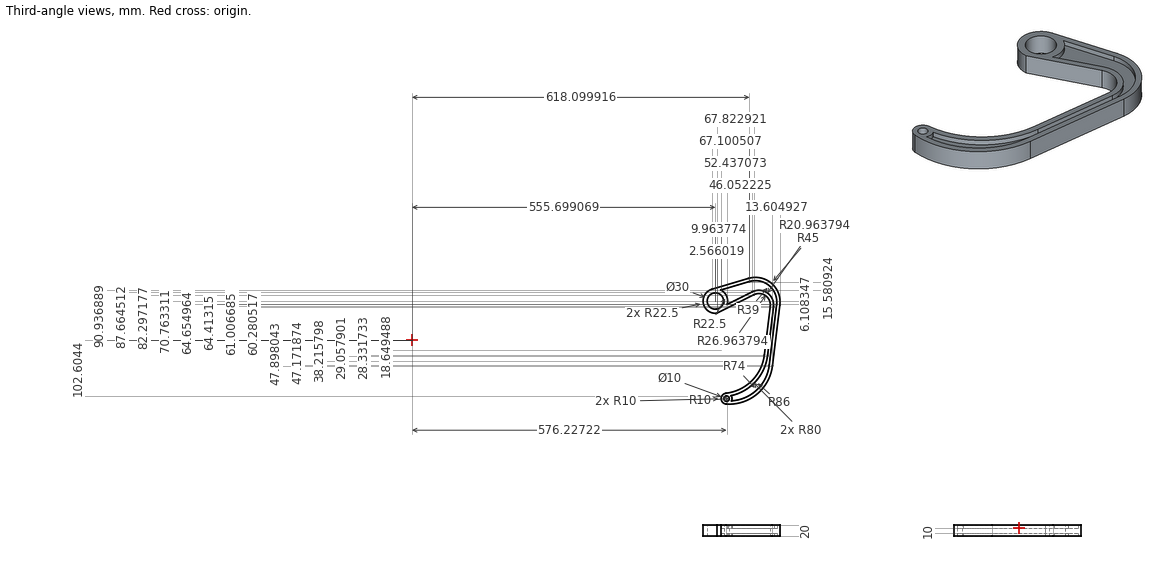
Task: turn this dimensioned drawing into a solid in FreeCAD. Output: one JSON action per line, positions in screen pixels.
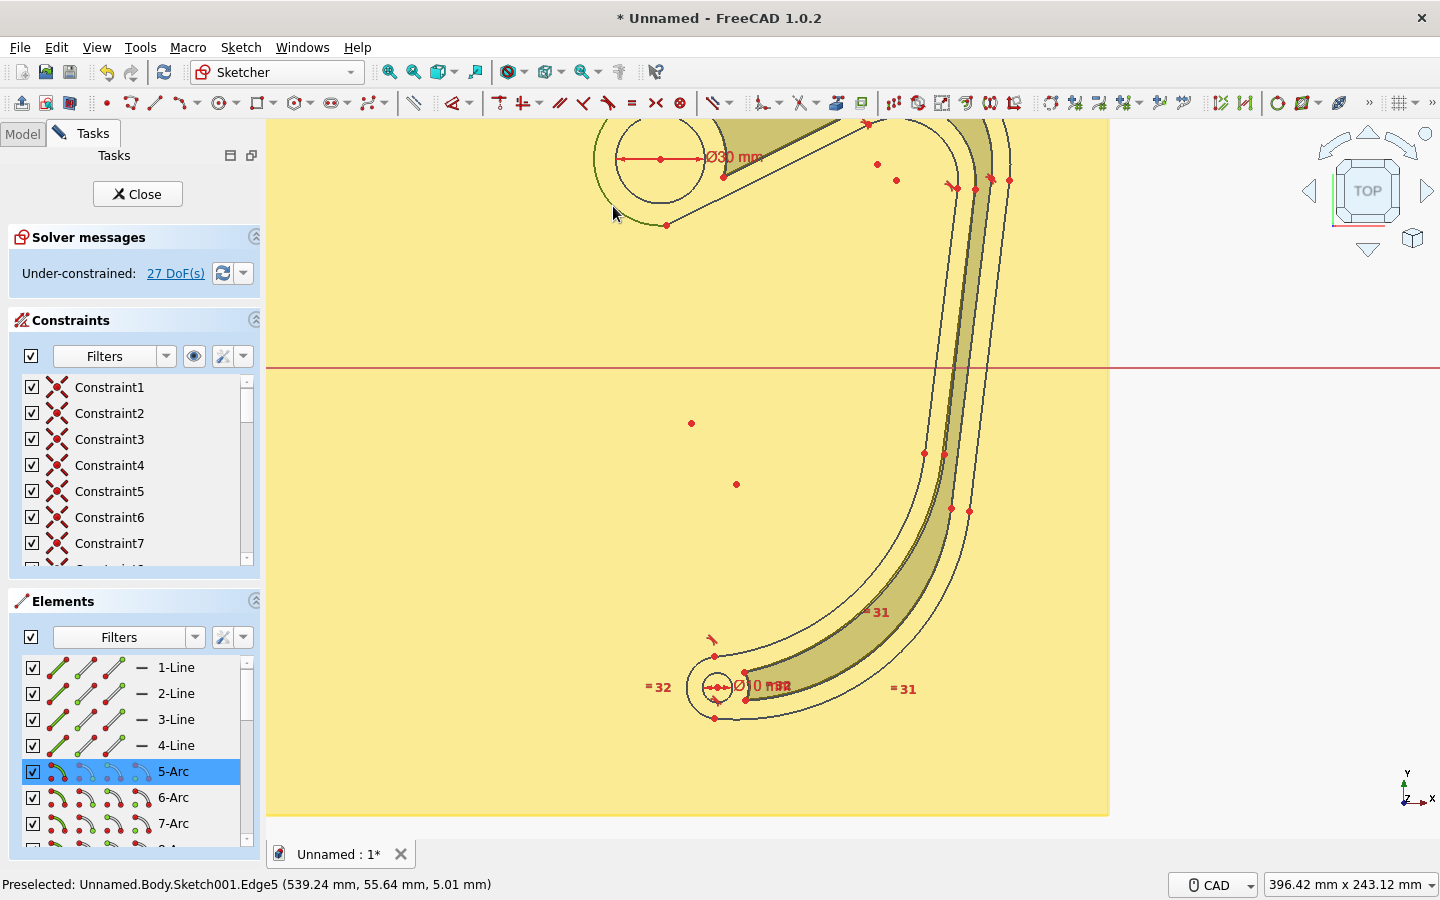
{"action": "left_click", "coordinate": [726, 150]}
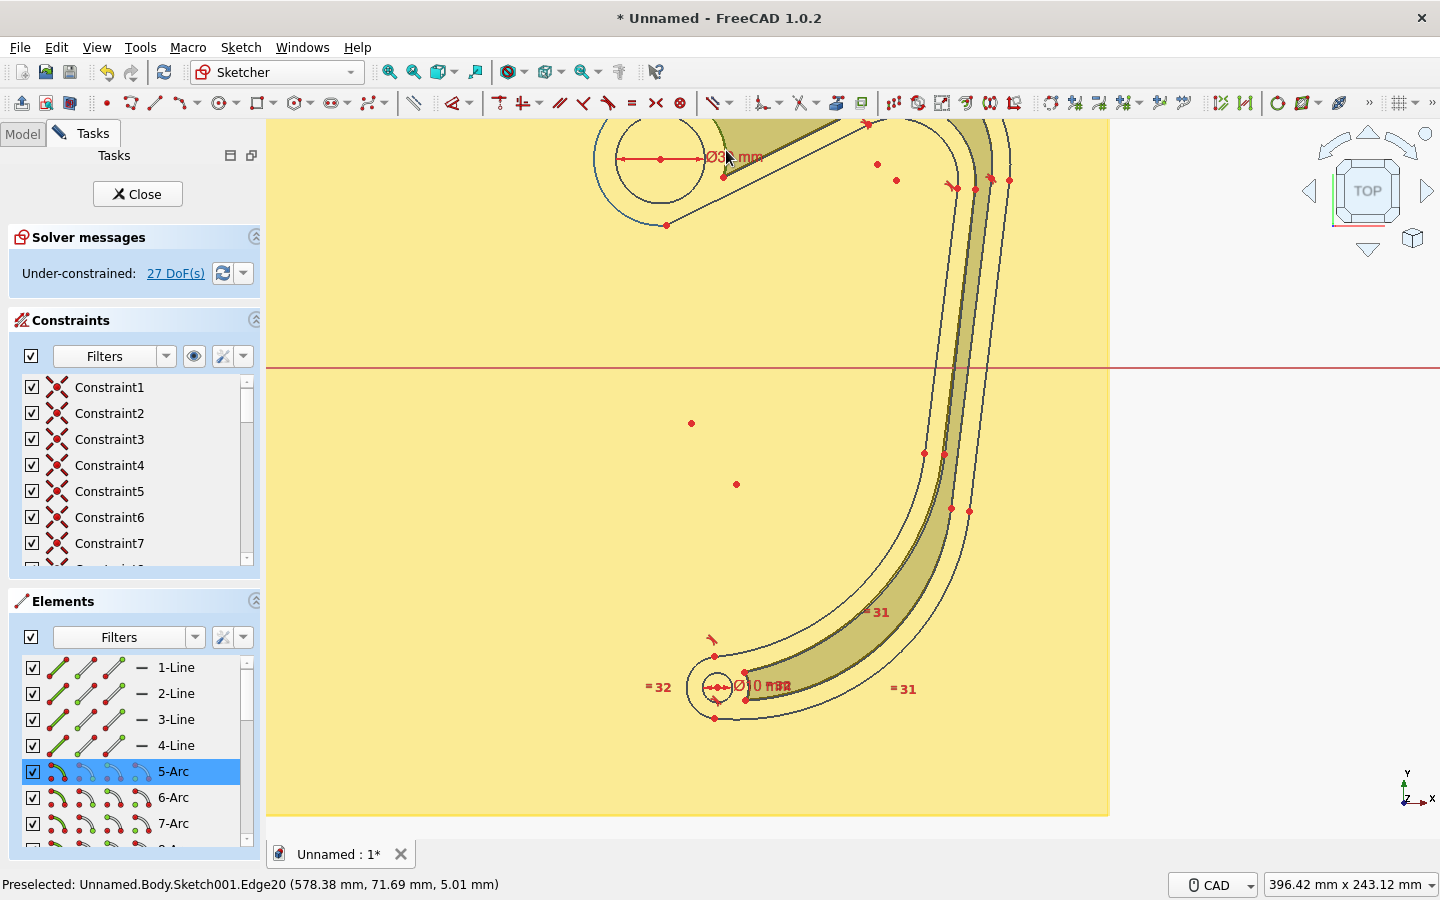
{"action": "key", "text": "e"}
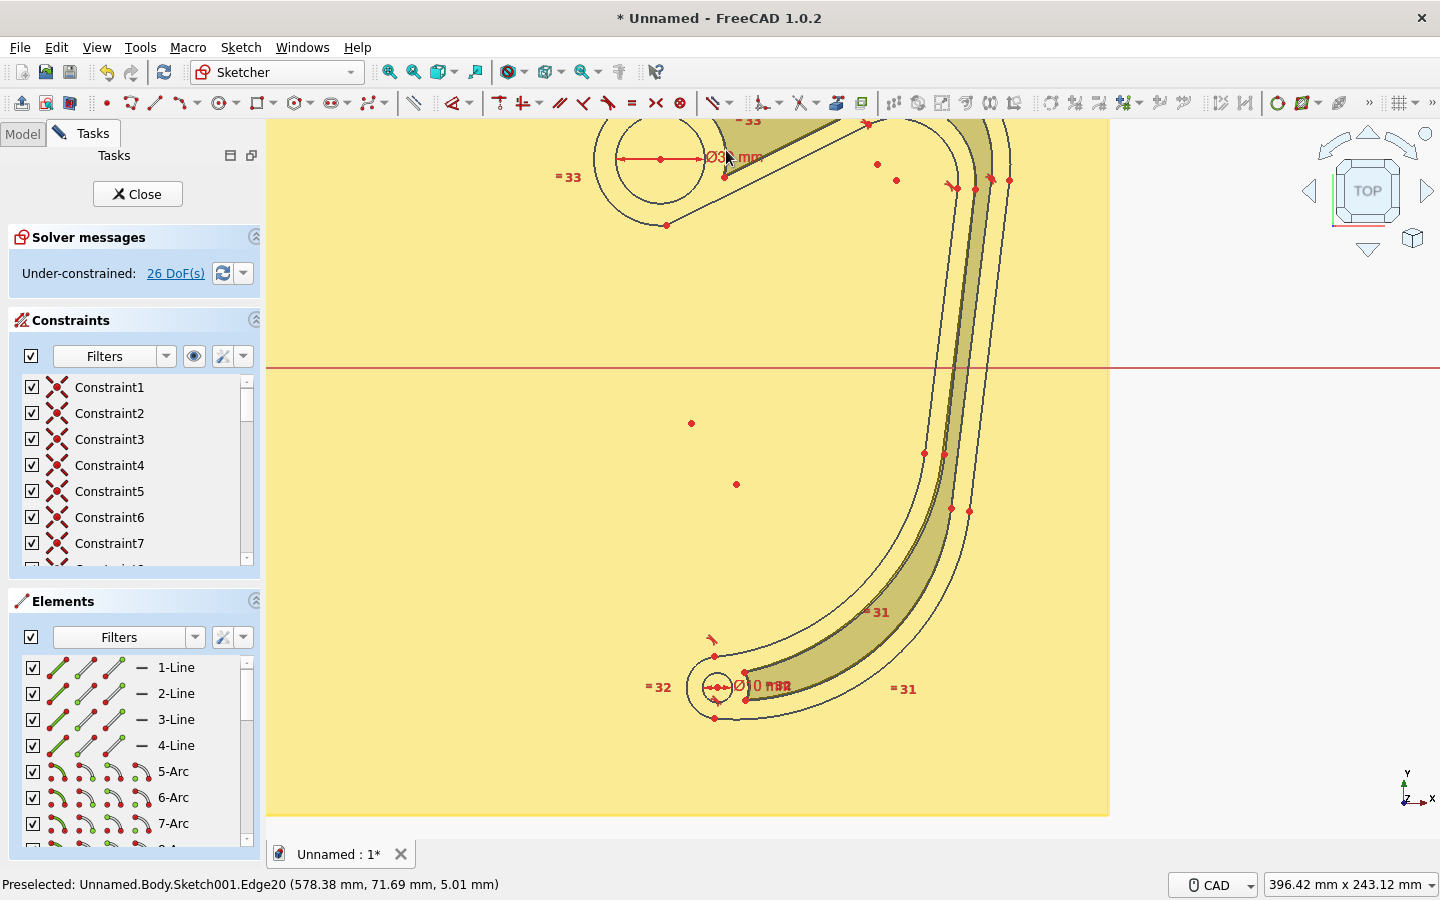
{"action": "left_click", "coordinate": [452, 104]}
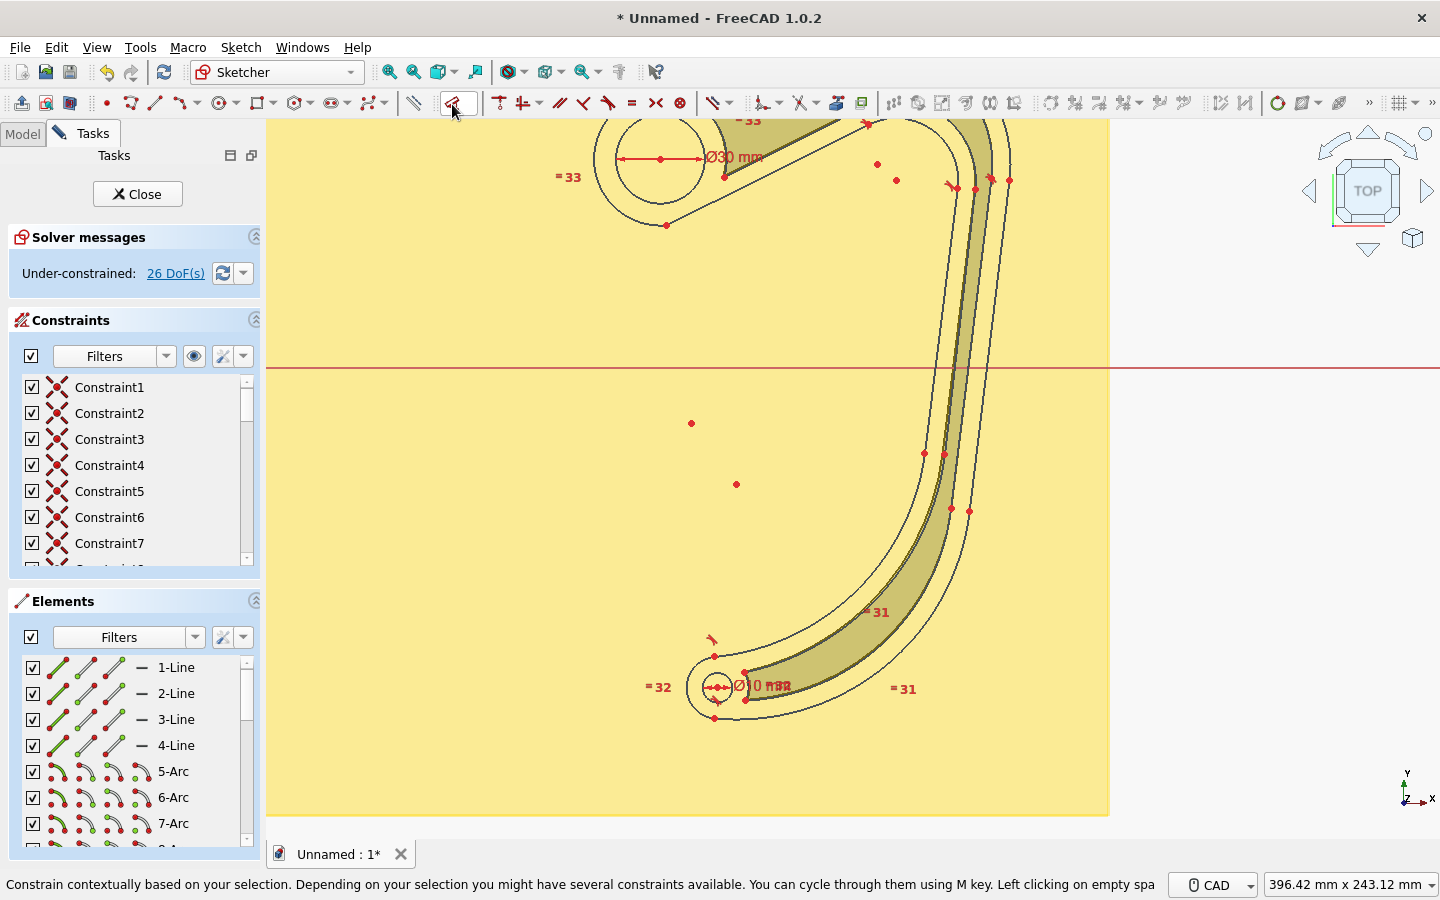
{"action": "left_click", "coordinate": [613, 206]}
{"action": "left_click", "coordinate": [590, 228]}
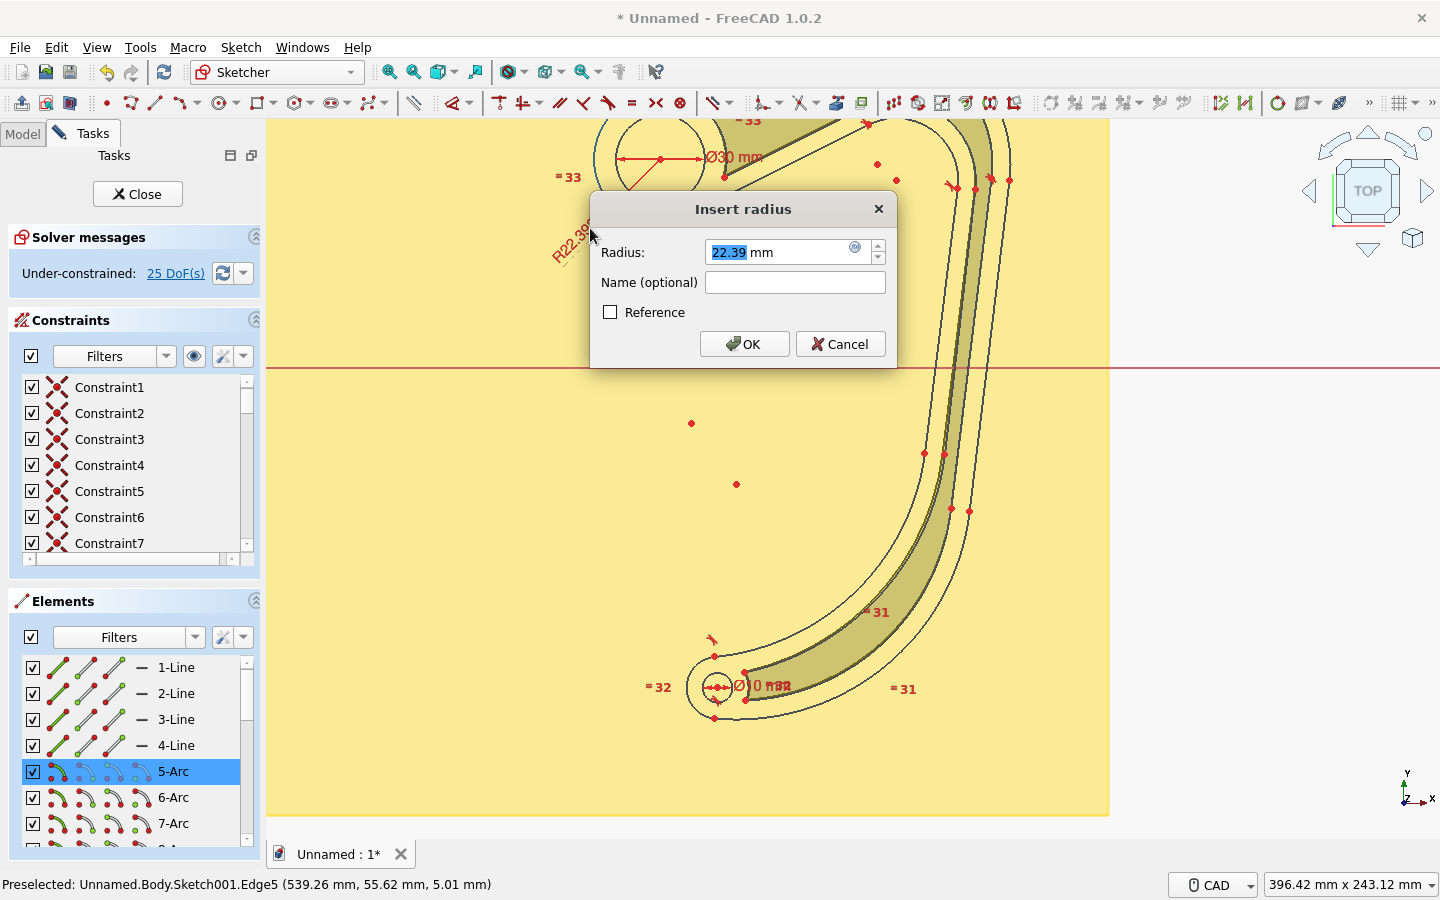
{"action": "type", "text": "22.5"}
{"action": "key", "text": "Return"}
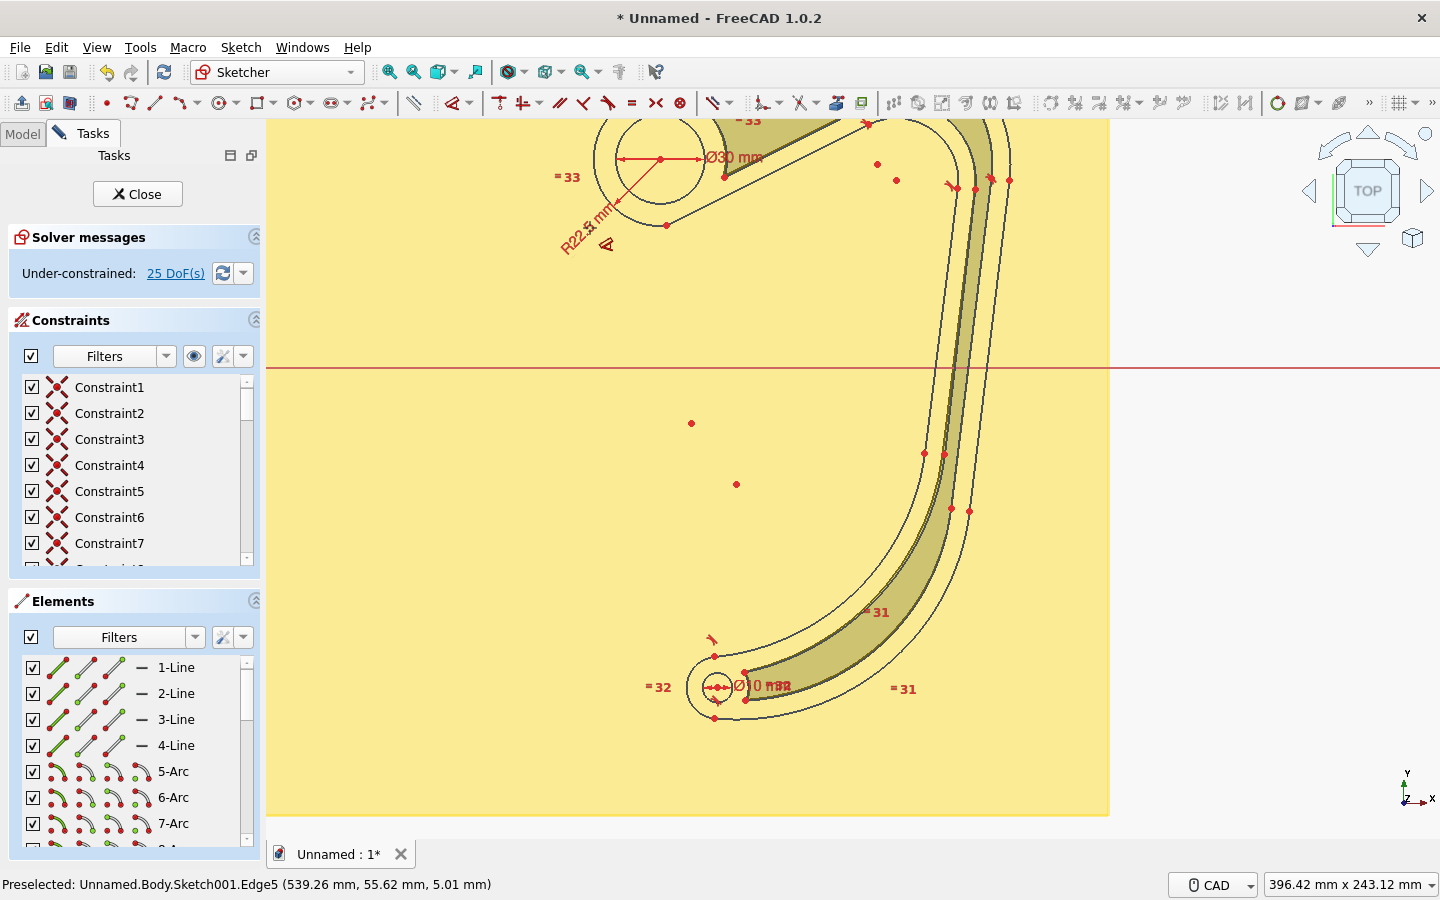
{"action": "left_click", "coordinate": [950, 149]}
{"action": "left_click", "coordinate": [815, 228]}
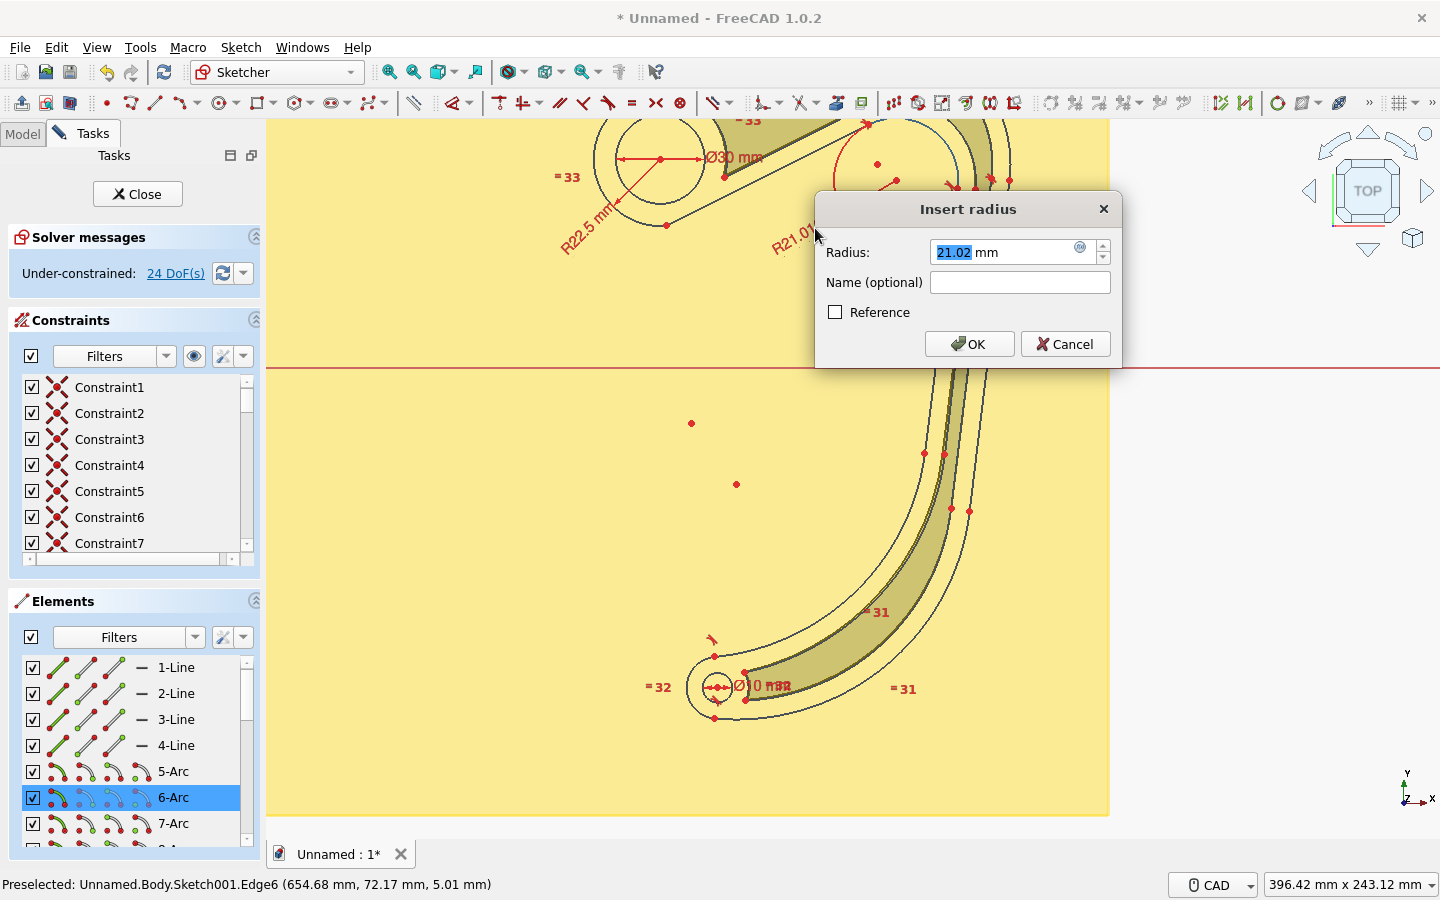
{"action": "type", "text": "20.963794"}
{"action": "key", "text": "Return"}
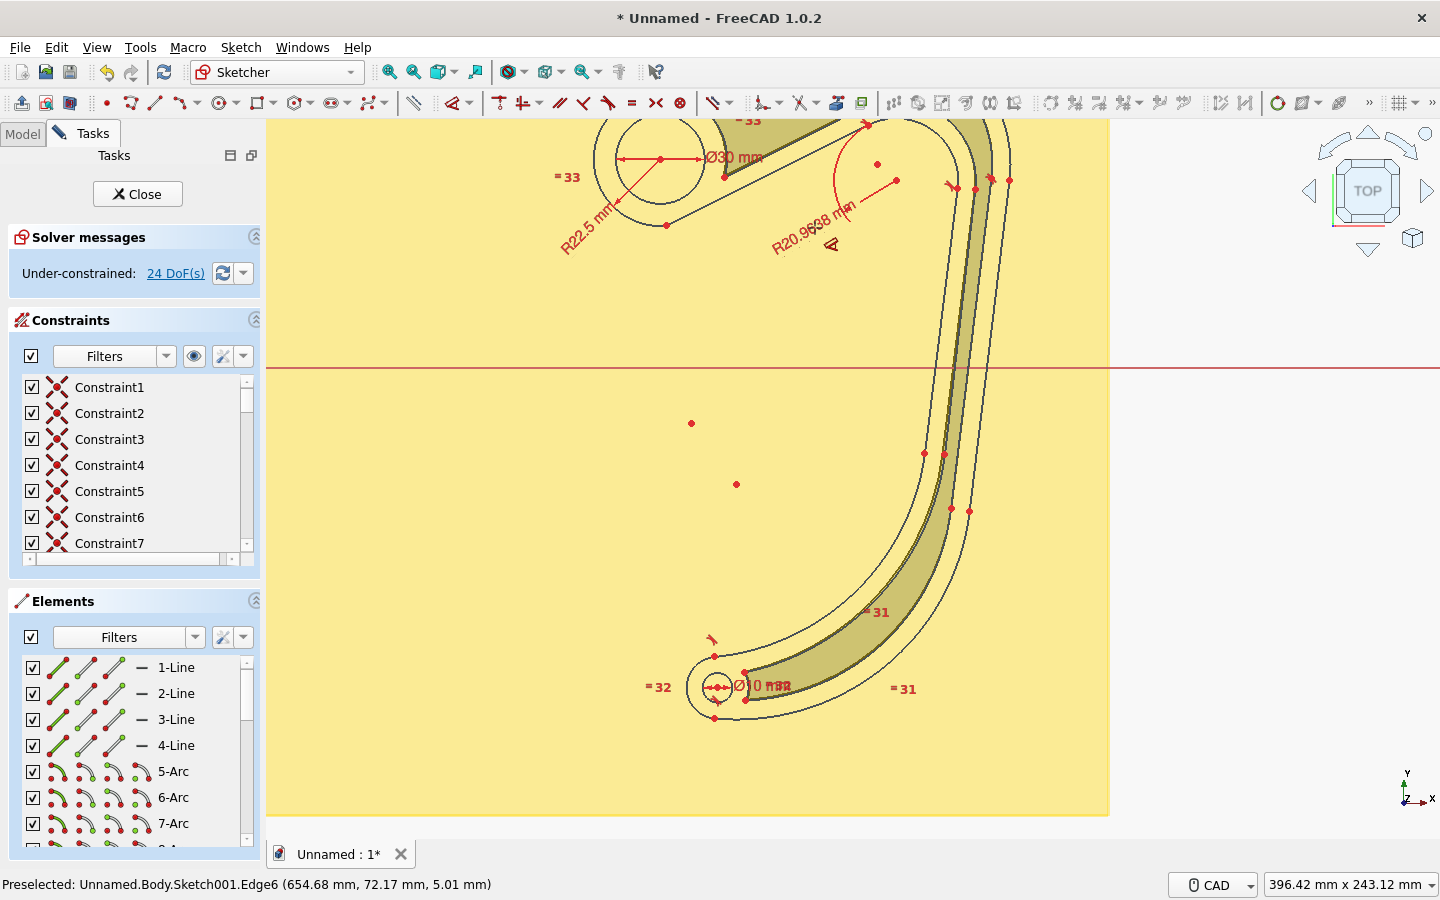
{"action": "left_click", "coordinate": [805, 629]}
{"action": "left_click", "coordinate": [564, 658]}